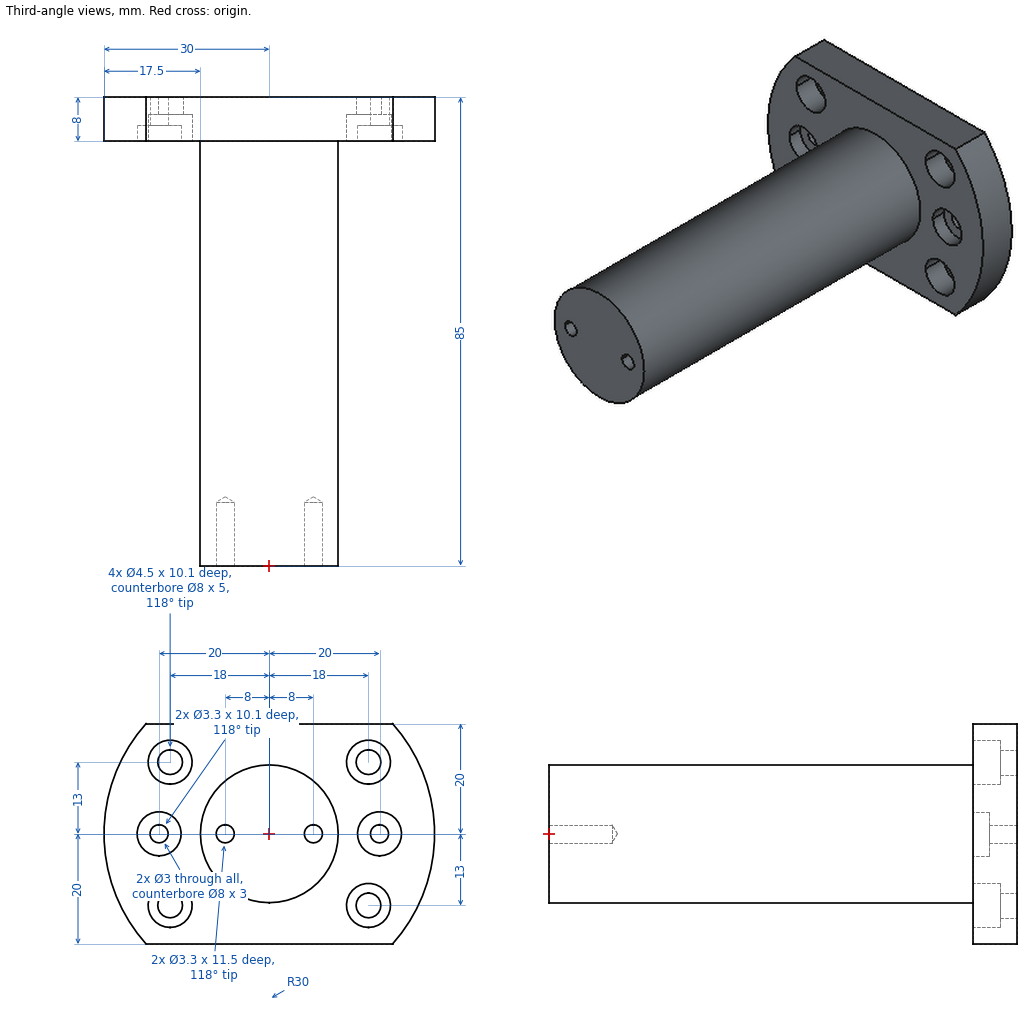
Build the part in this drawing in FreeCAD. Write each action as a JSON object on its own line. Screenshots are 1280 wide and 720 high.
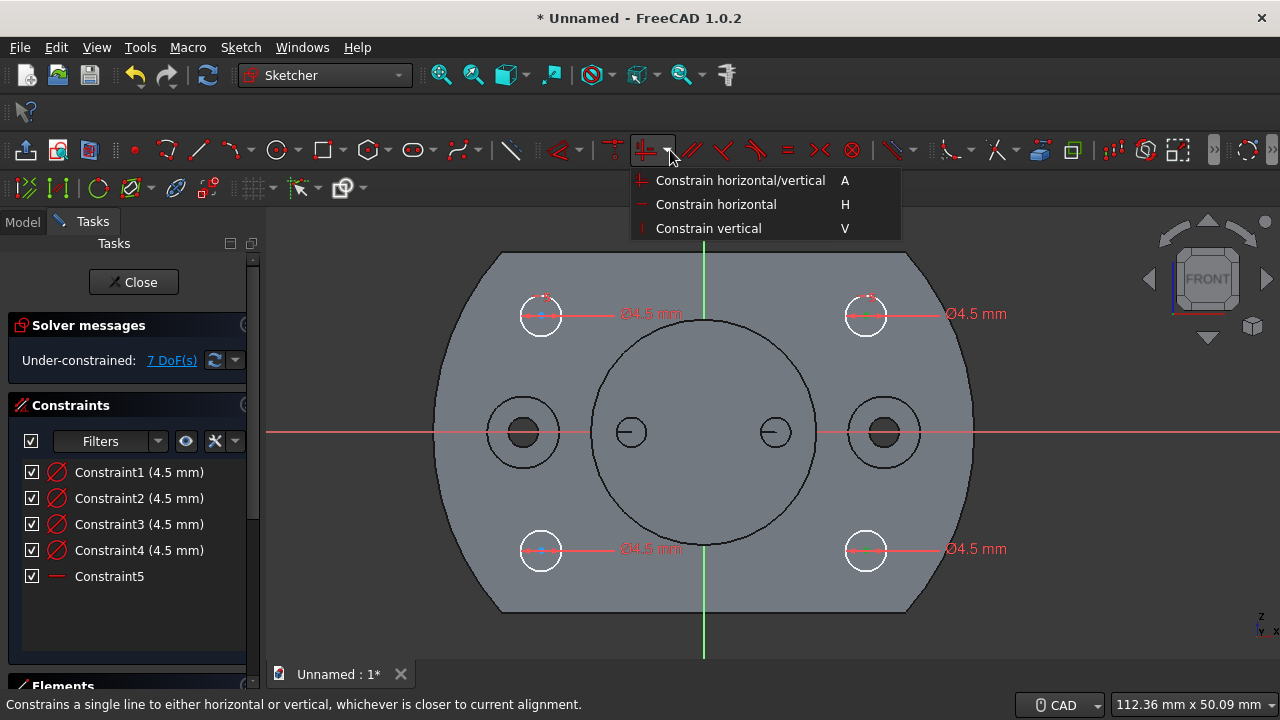
{"action": "left_click", "coordinate": [766, 228]}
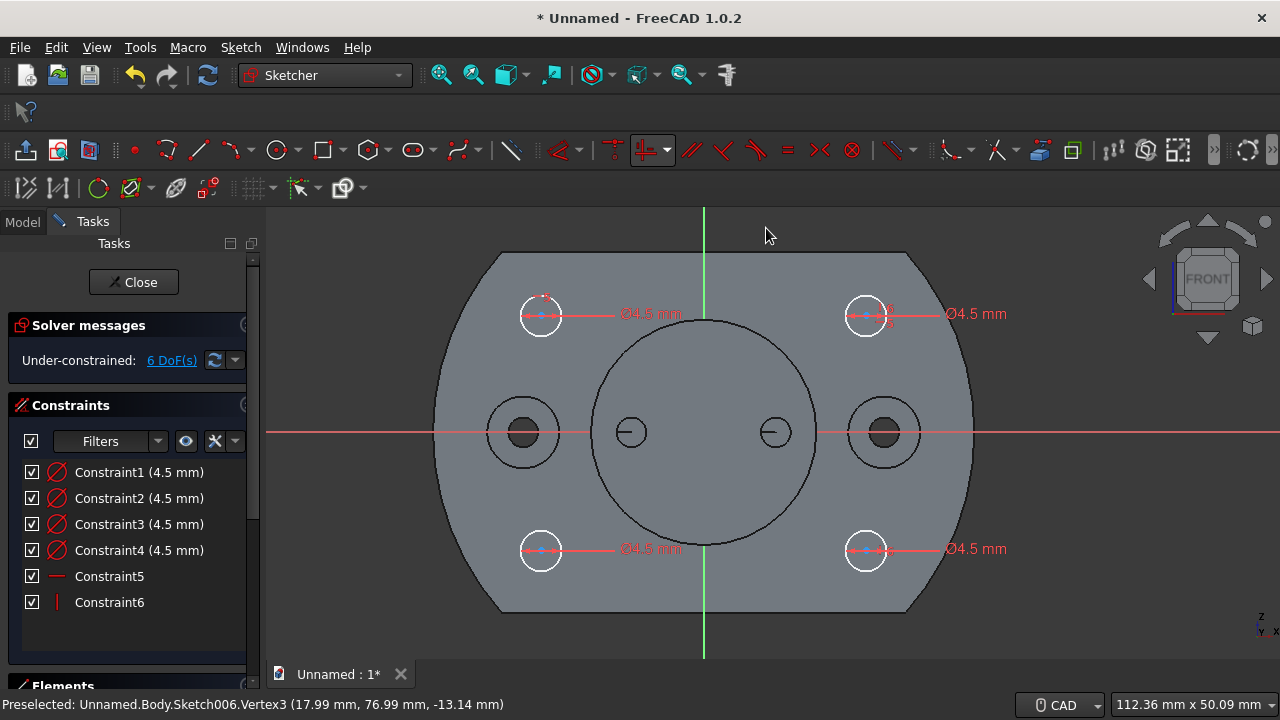
{"action": "left_click", "coordinate": [541, 316]}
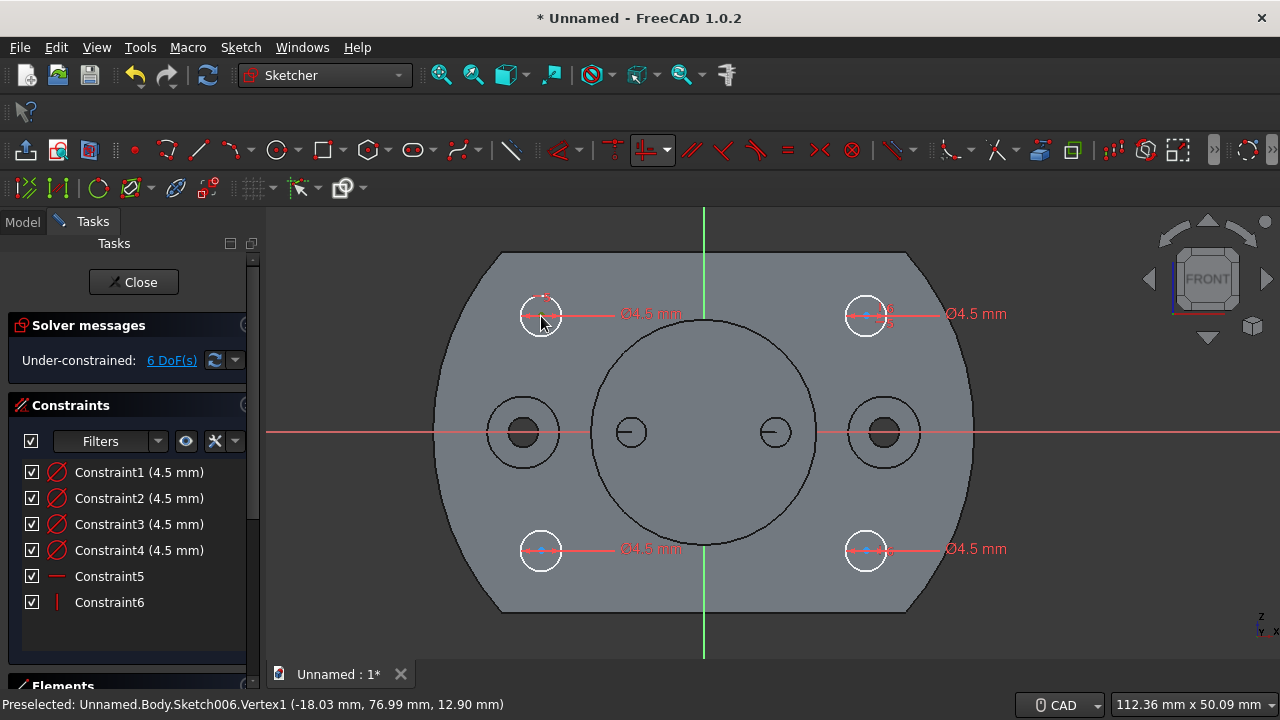
{"action": "left_click", "coordinate": [541, 551]}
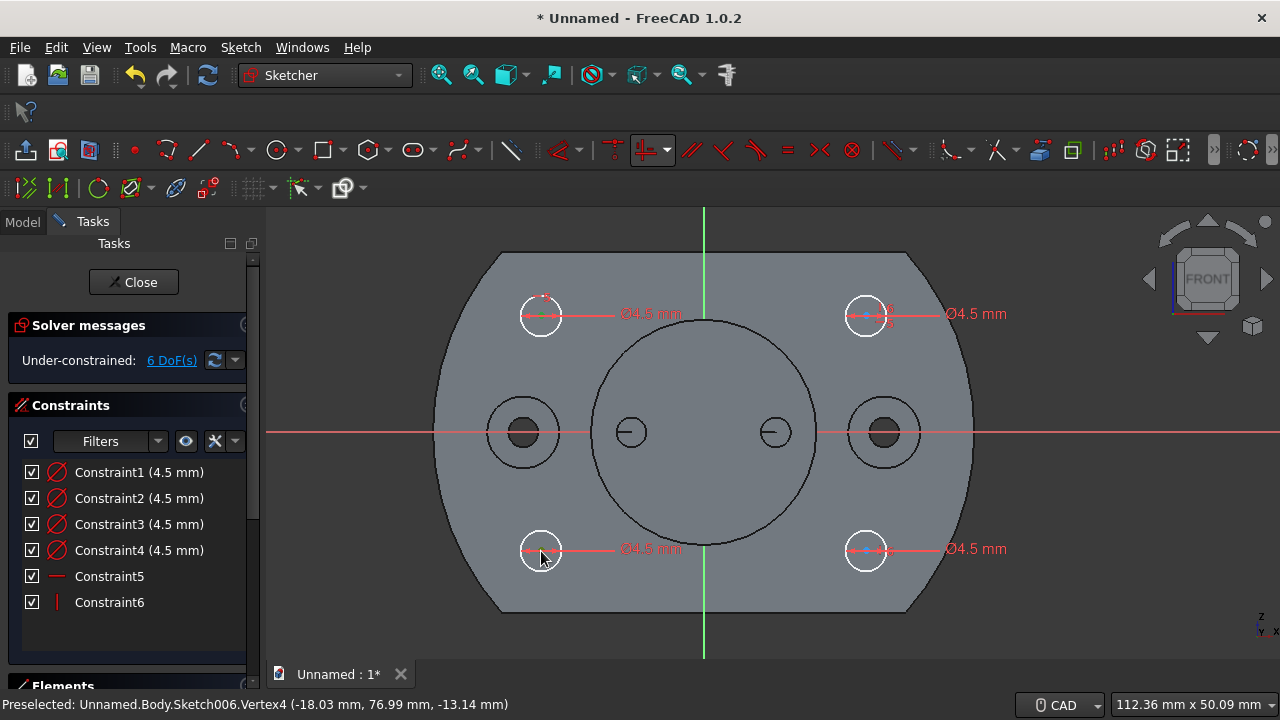
{"action": "key", "text": "v"}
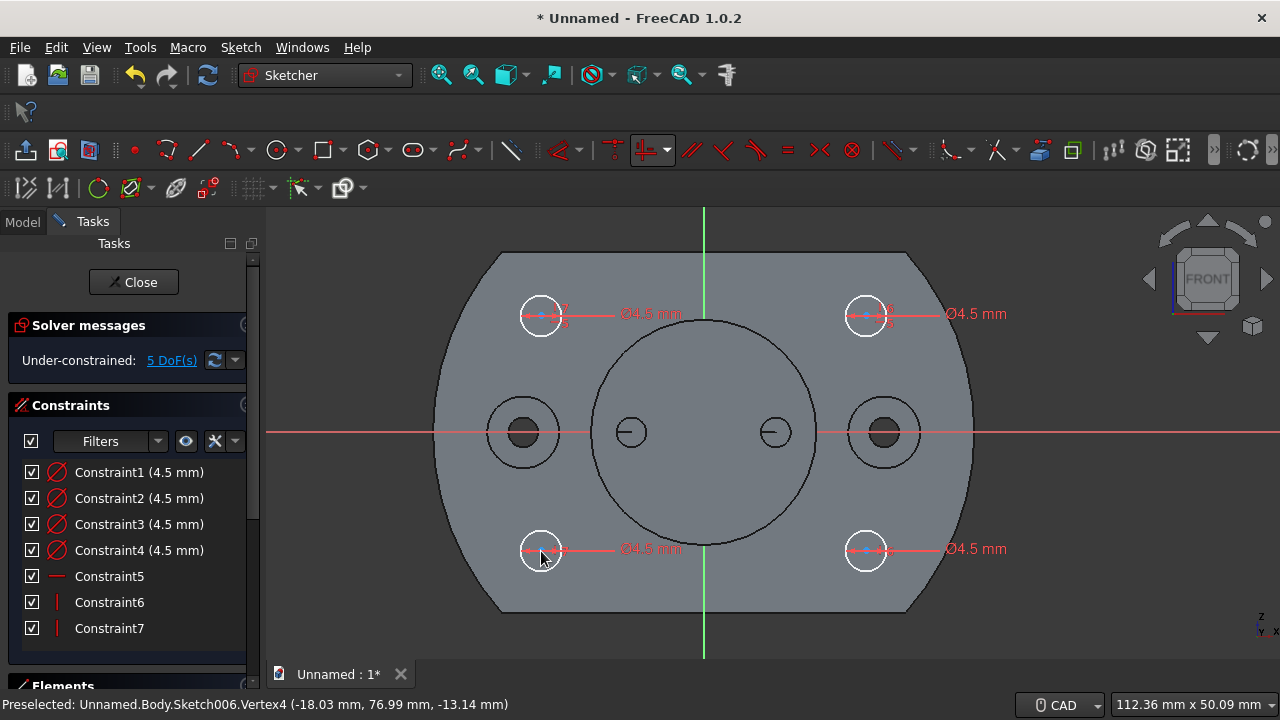
{"action": "left_click", "coordinate": [866, 551]}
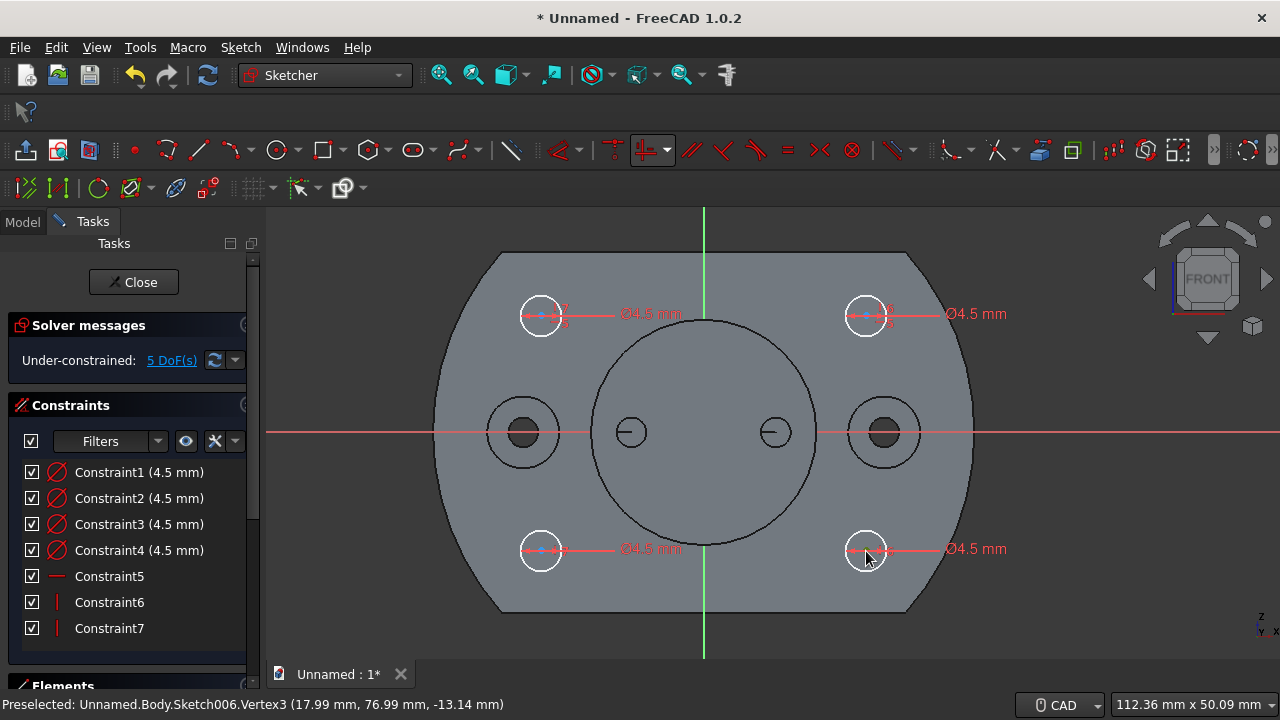
{"action": "left_click", "coordinate": [541, 551]}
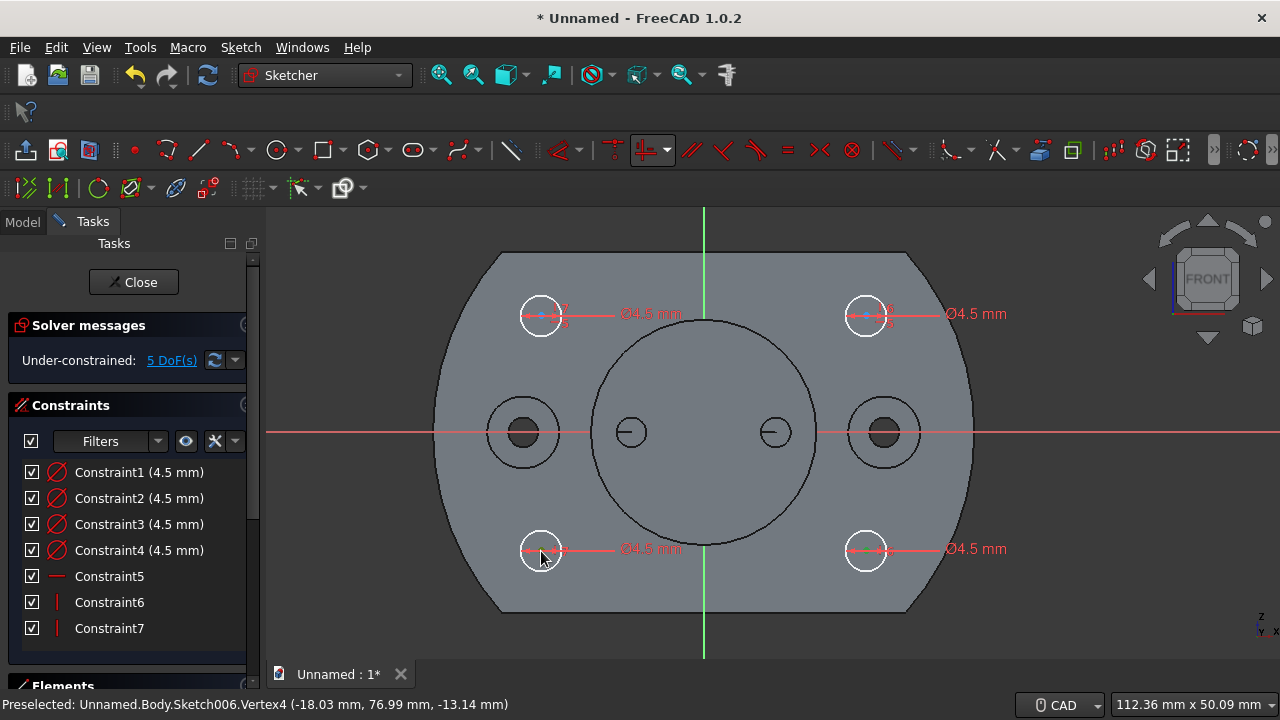
{"action": "left_click", "coordinate": [670, 150]}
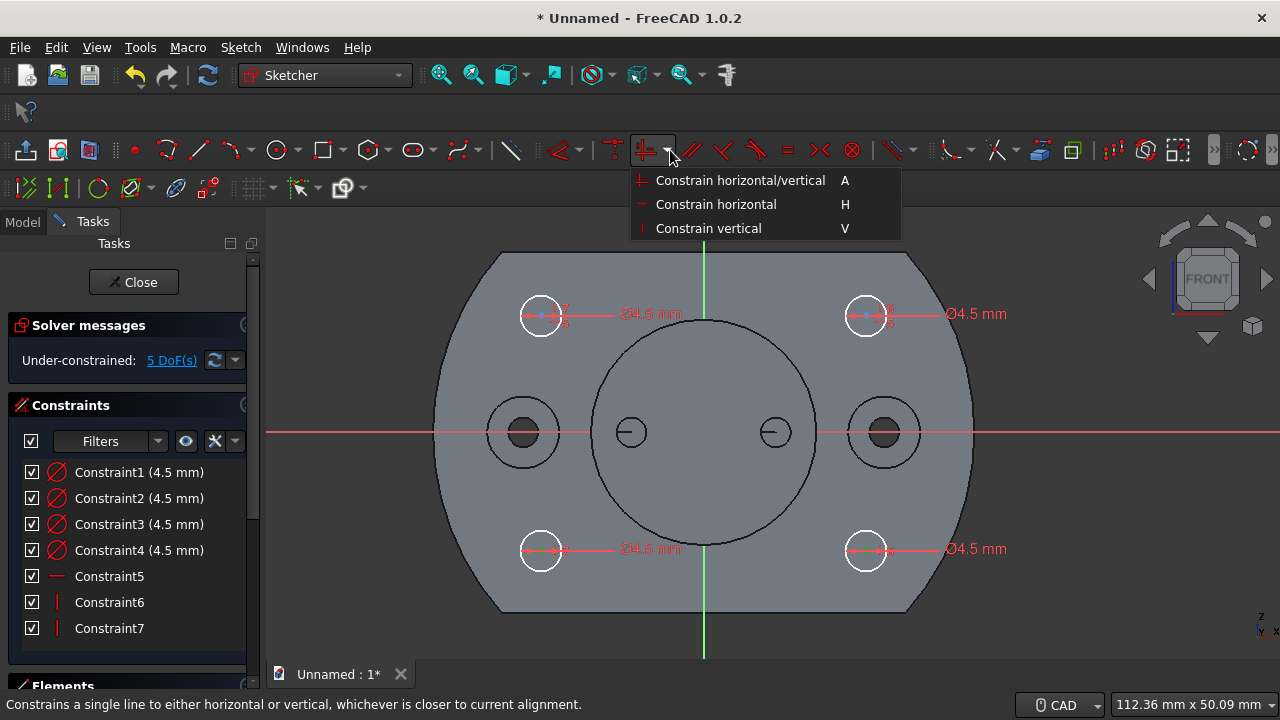
{"action": "left_click", "coordinate": [766, 204]}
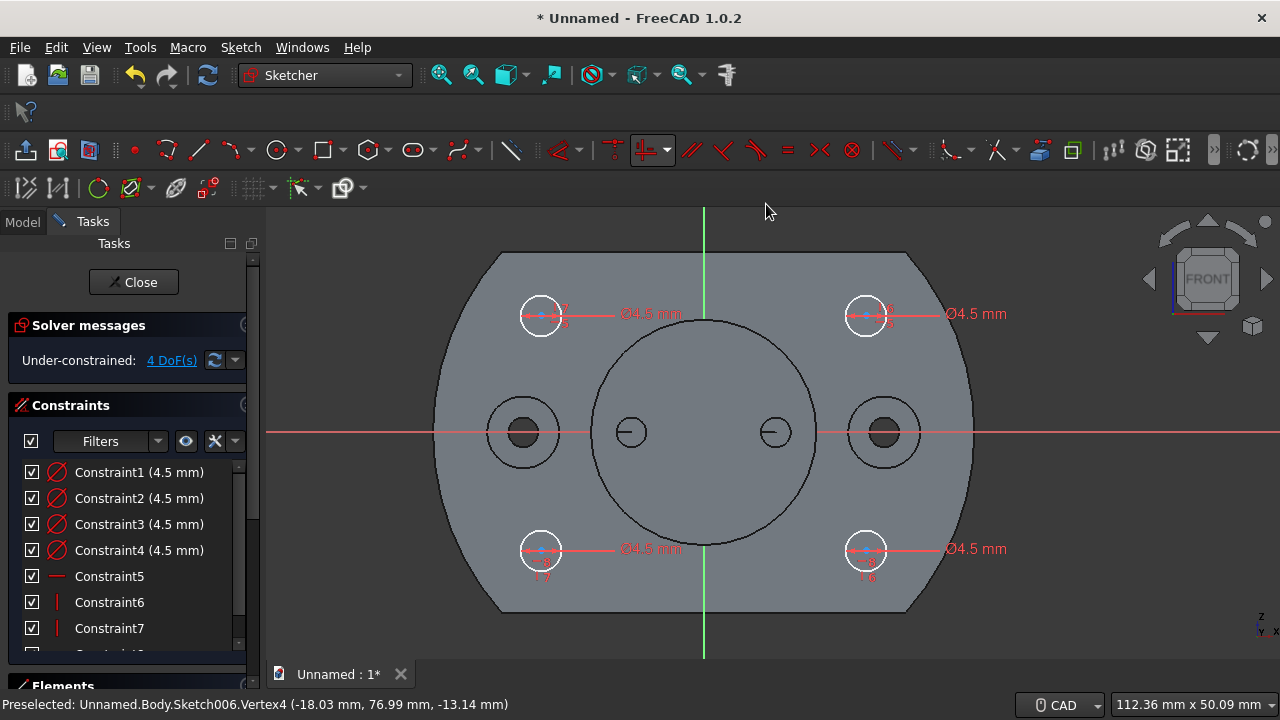
{"action": "left_click", "coordinate": [558, 150]}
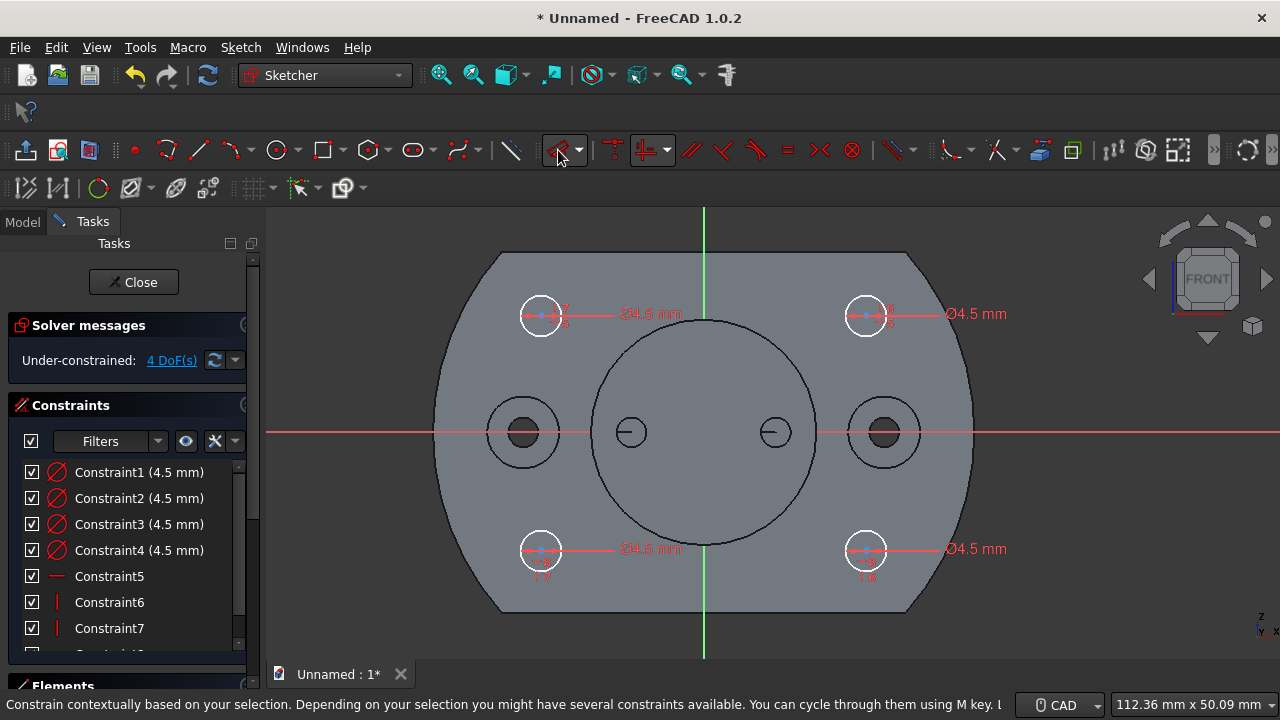
{"action": "left_click", "coordinate": [541, 316]}
{"action": "left_click", "coordinate": [622, 282]}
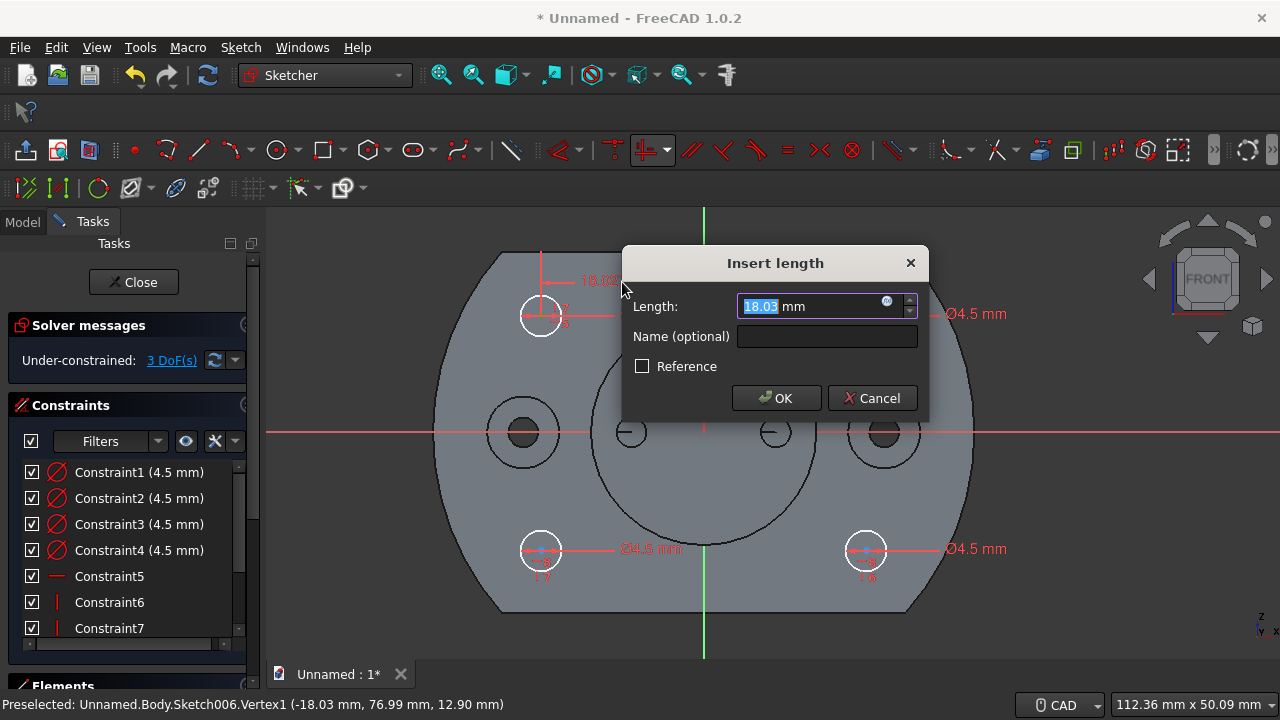
{"action": "type", "text": "18"}
{"action": "key", "text": "Return"}